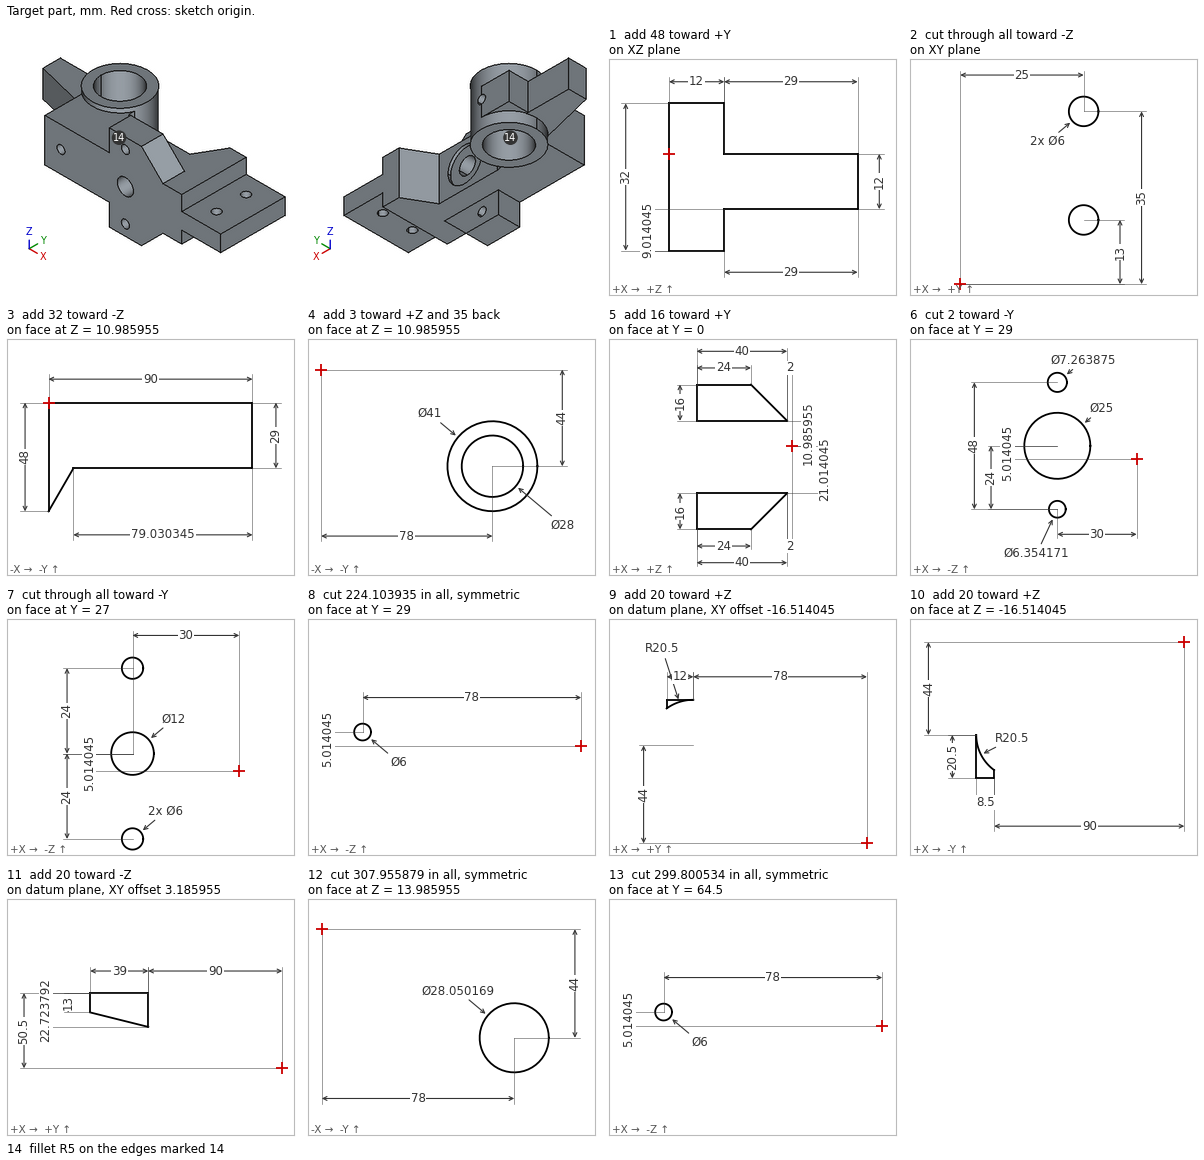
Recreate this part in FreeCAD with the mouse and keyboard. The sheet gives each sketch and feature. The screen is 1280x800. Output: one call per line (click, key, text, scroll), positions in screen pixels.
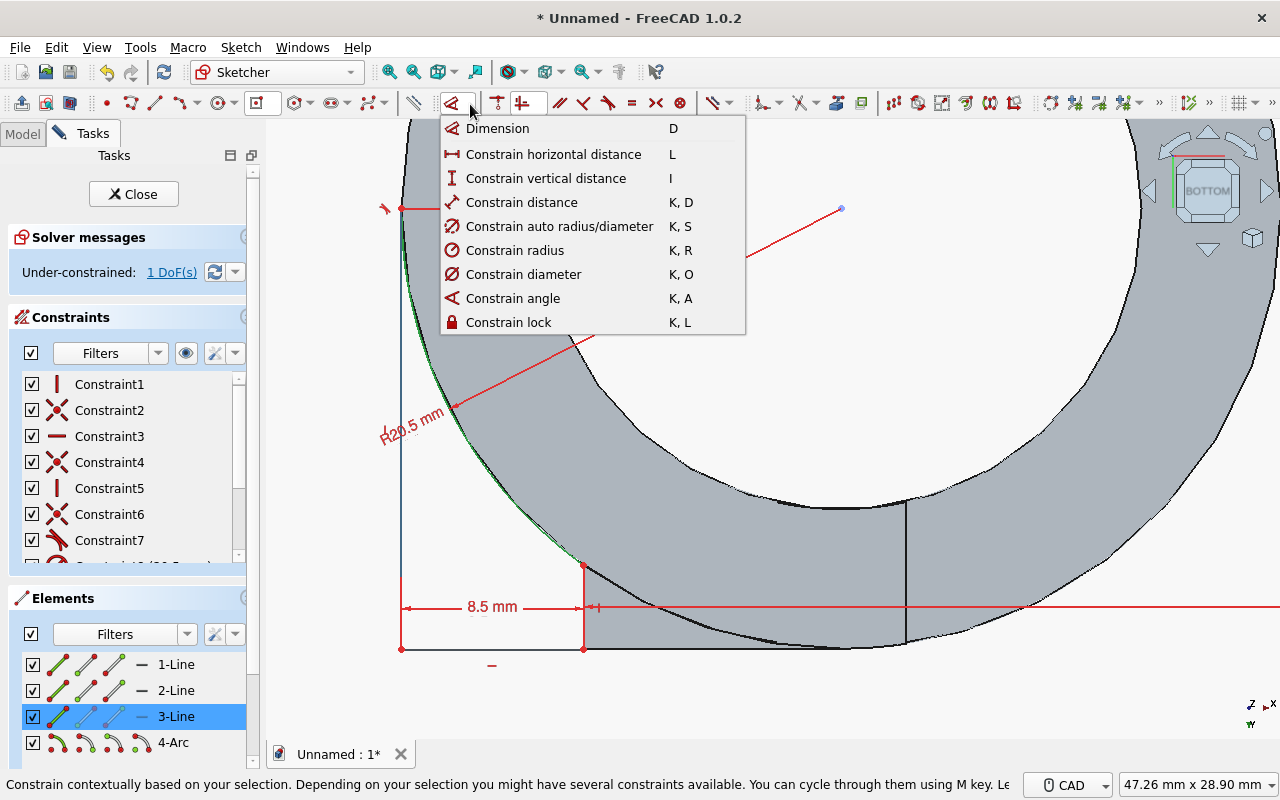
click(593, 178)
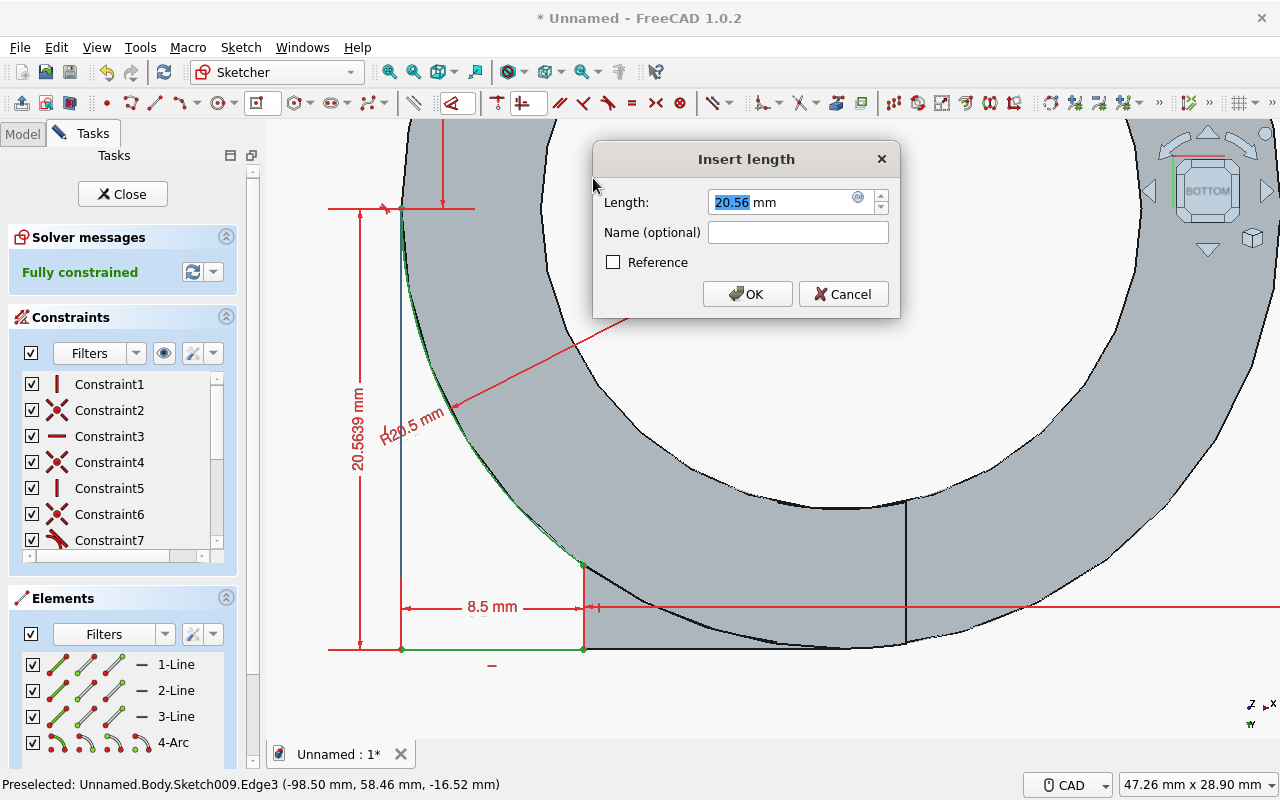
text(20.5)
key(Return)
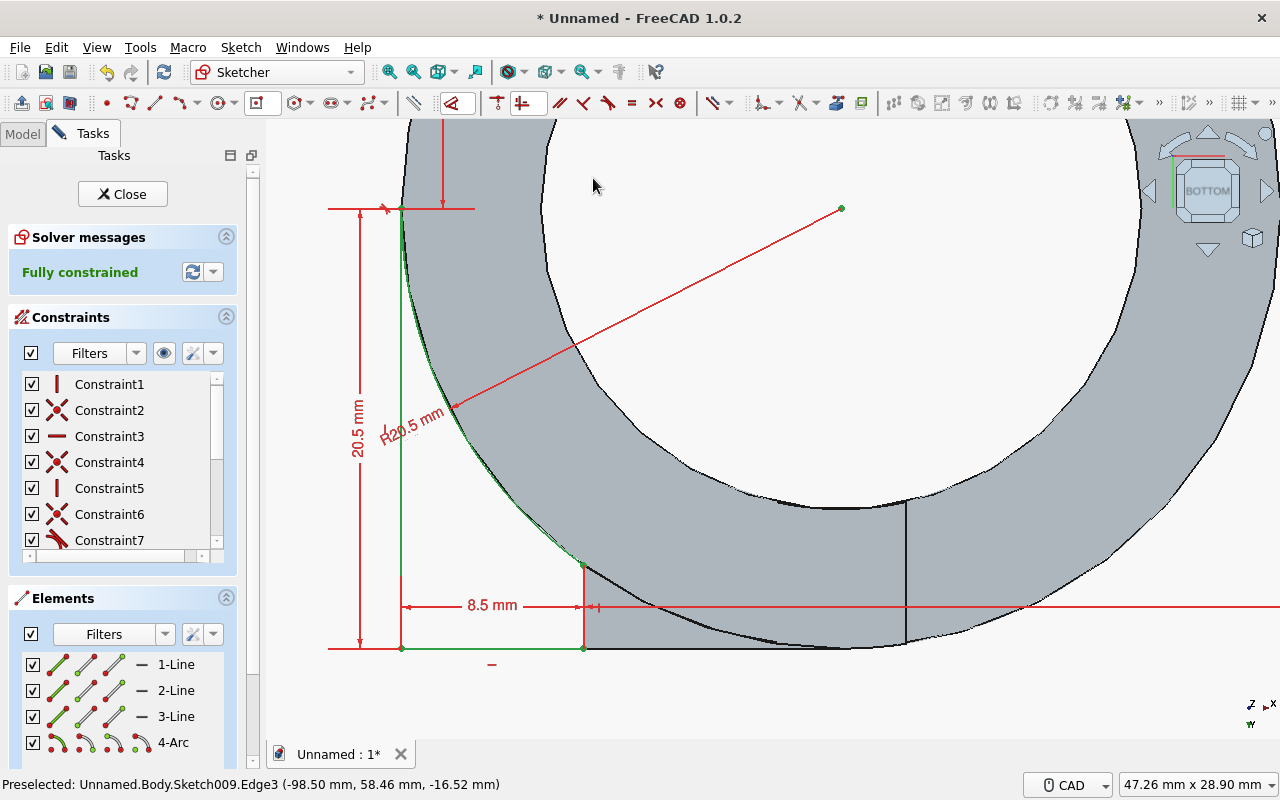
click(123, 194)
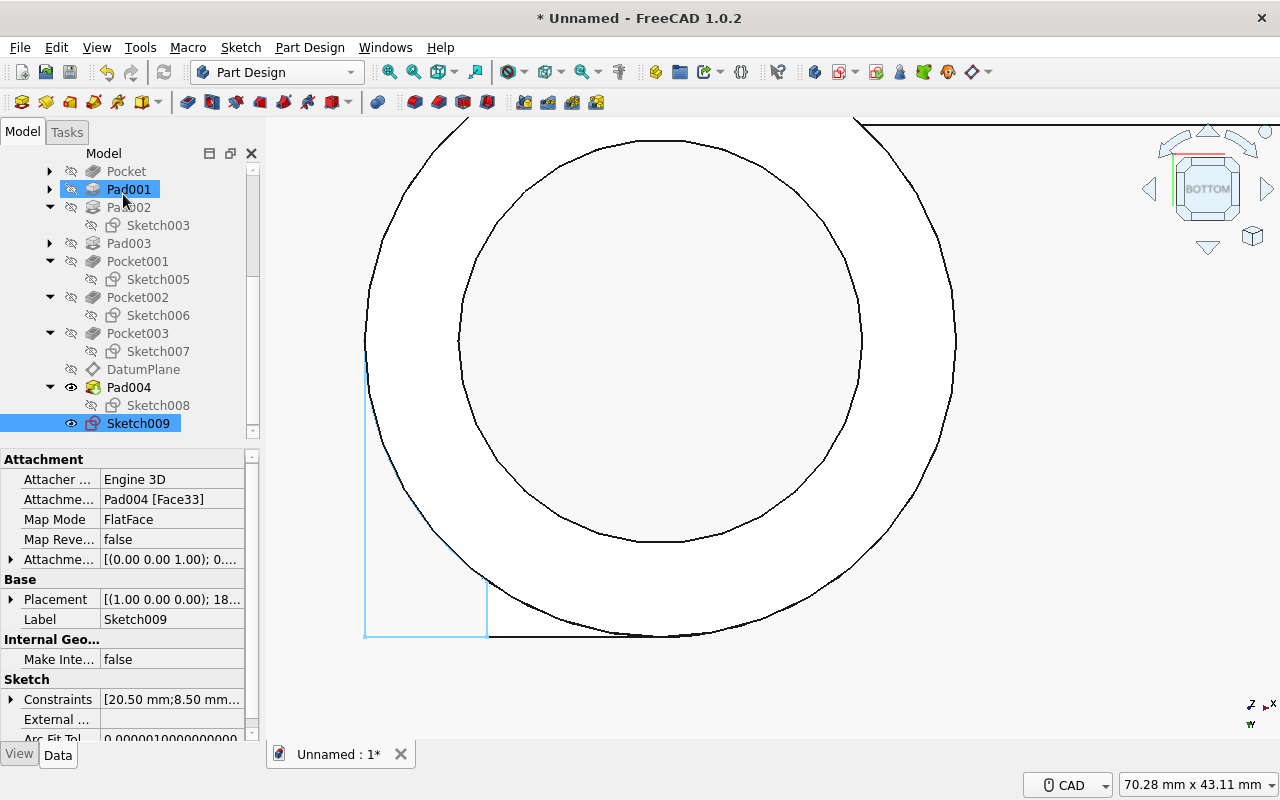
click(22, 102)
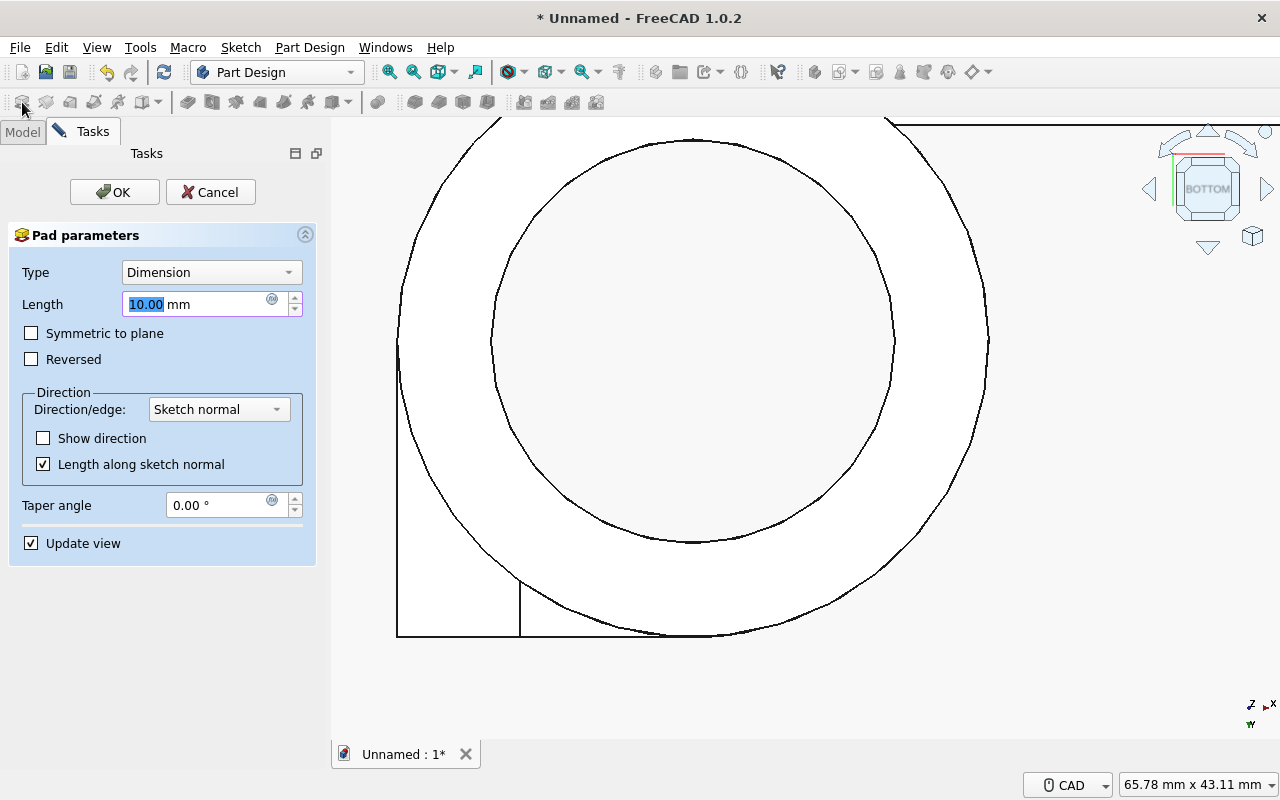
text(20)
key(Tab)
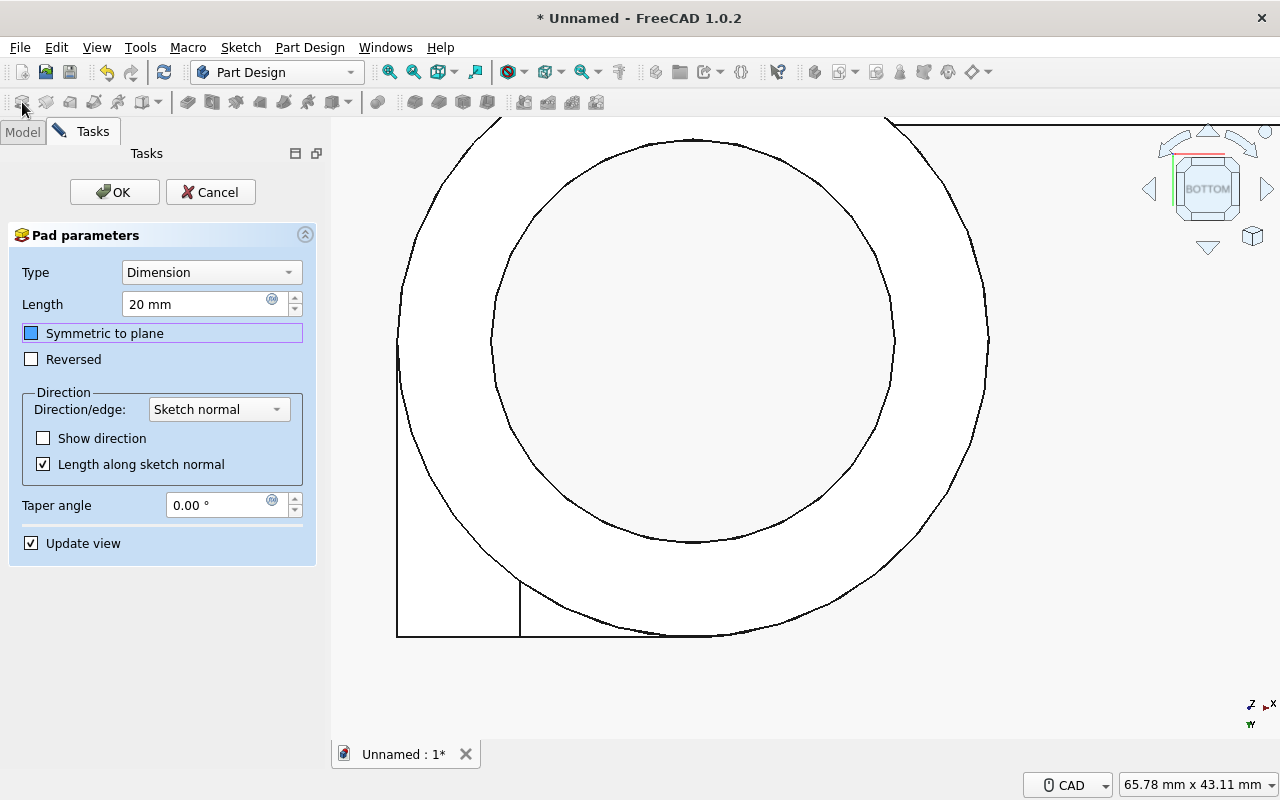
click(30, 359)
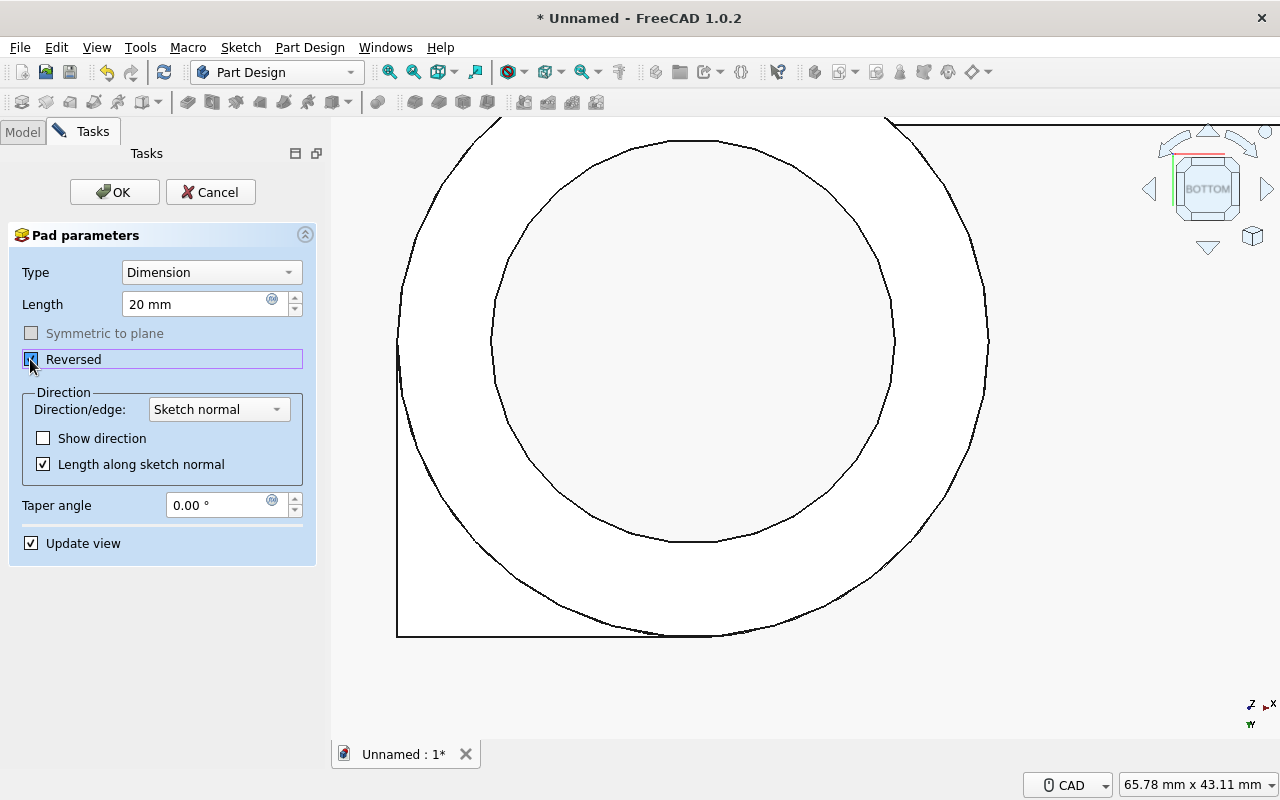
click(115, 192)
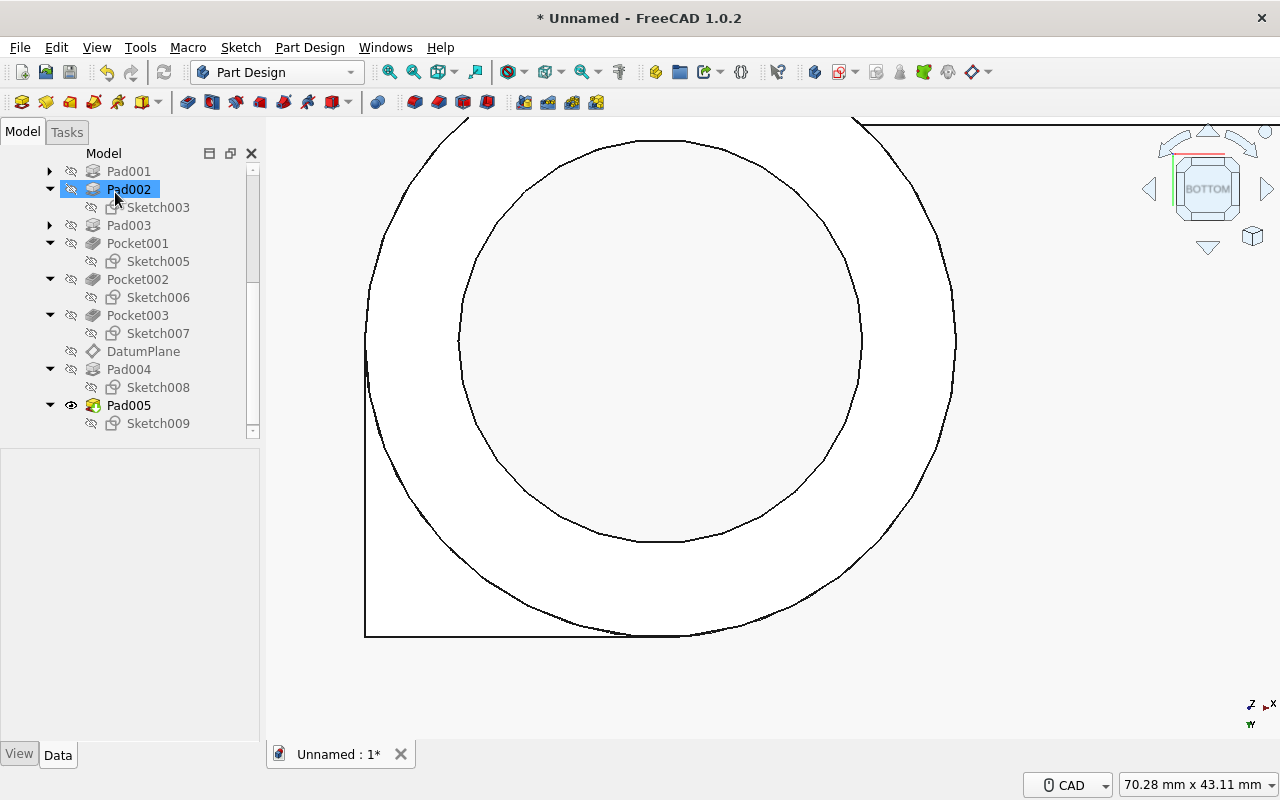
key(v)
key(f)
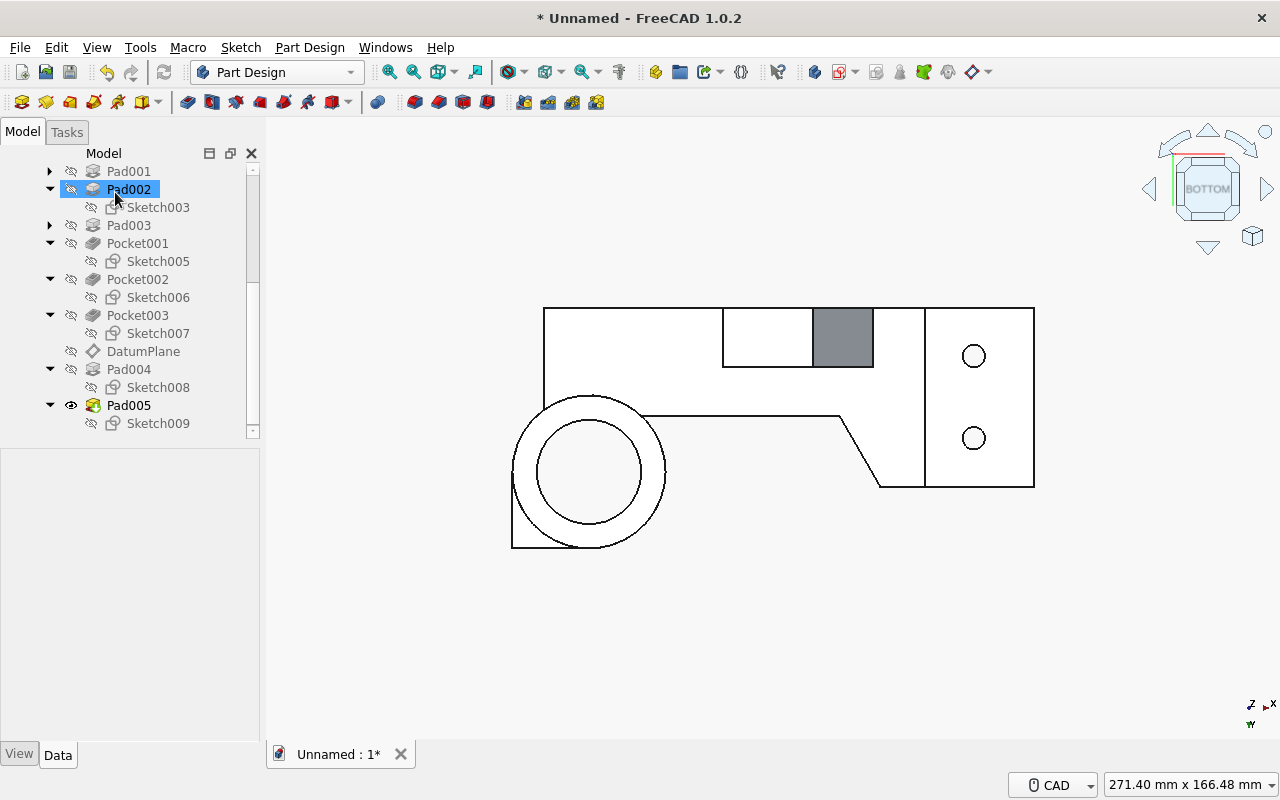
scroll(140, 293, down, 3)